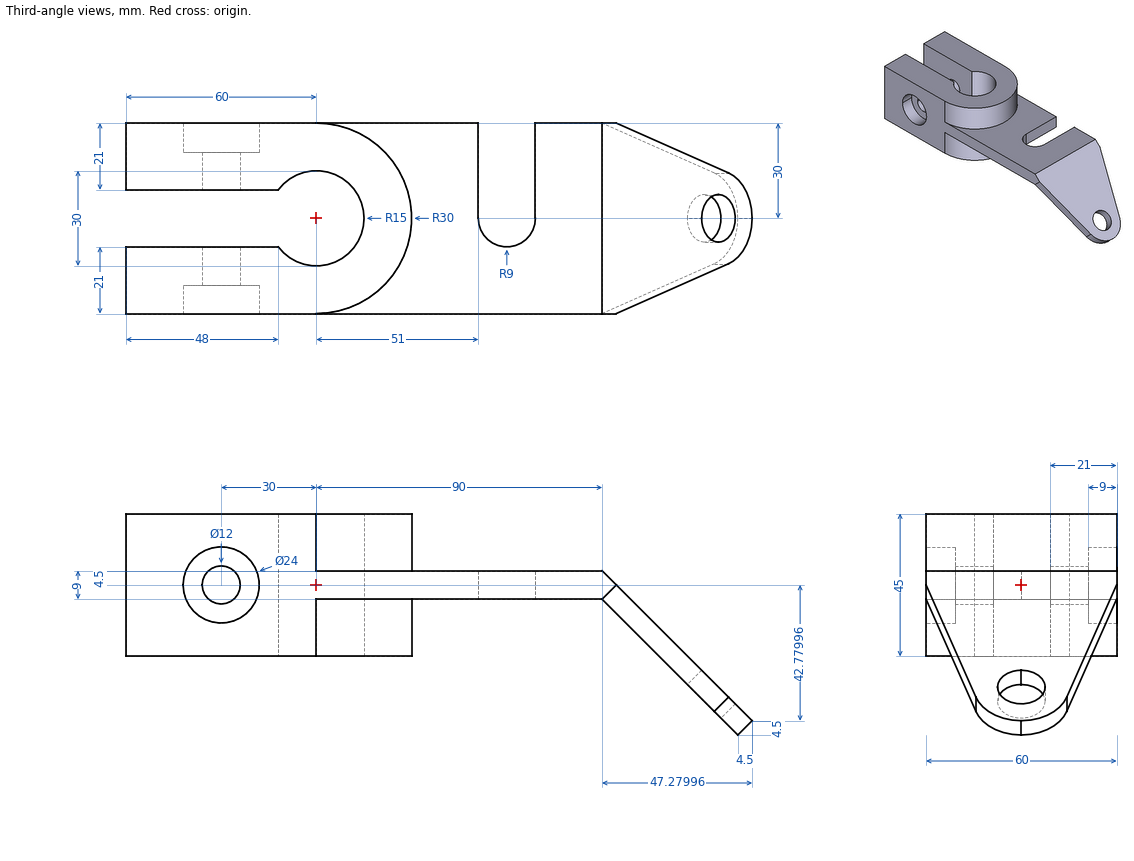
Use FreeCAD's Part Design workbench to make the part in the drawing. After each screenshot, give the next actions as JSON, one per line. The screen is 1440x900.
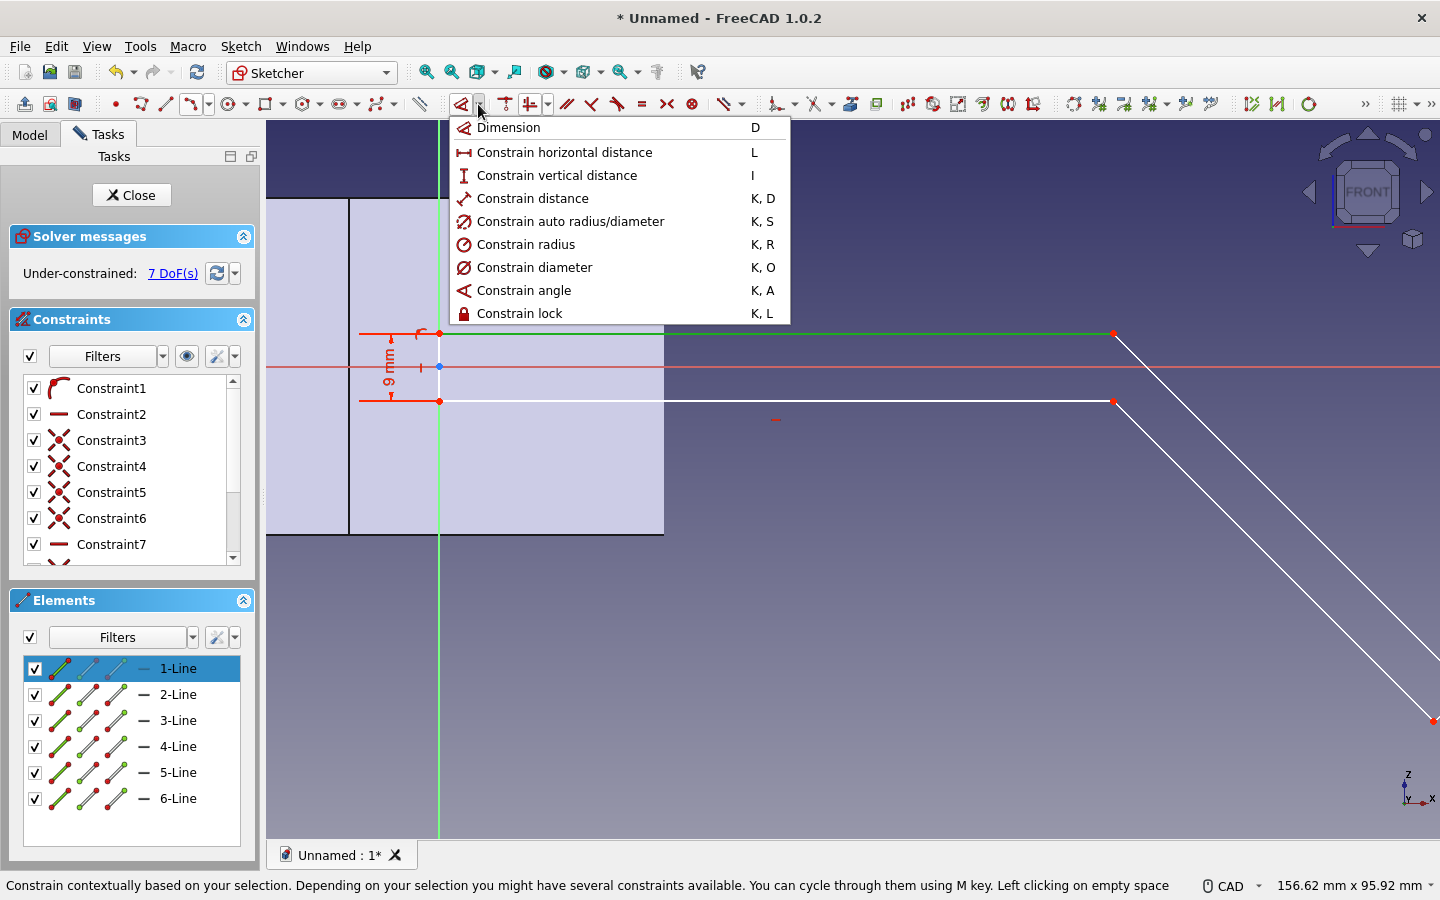
{"action": "left_click", "coordinate": [620, 152]}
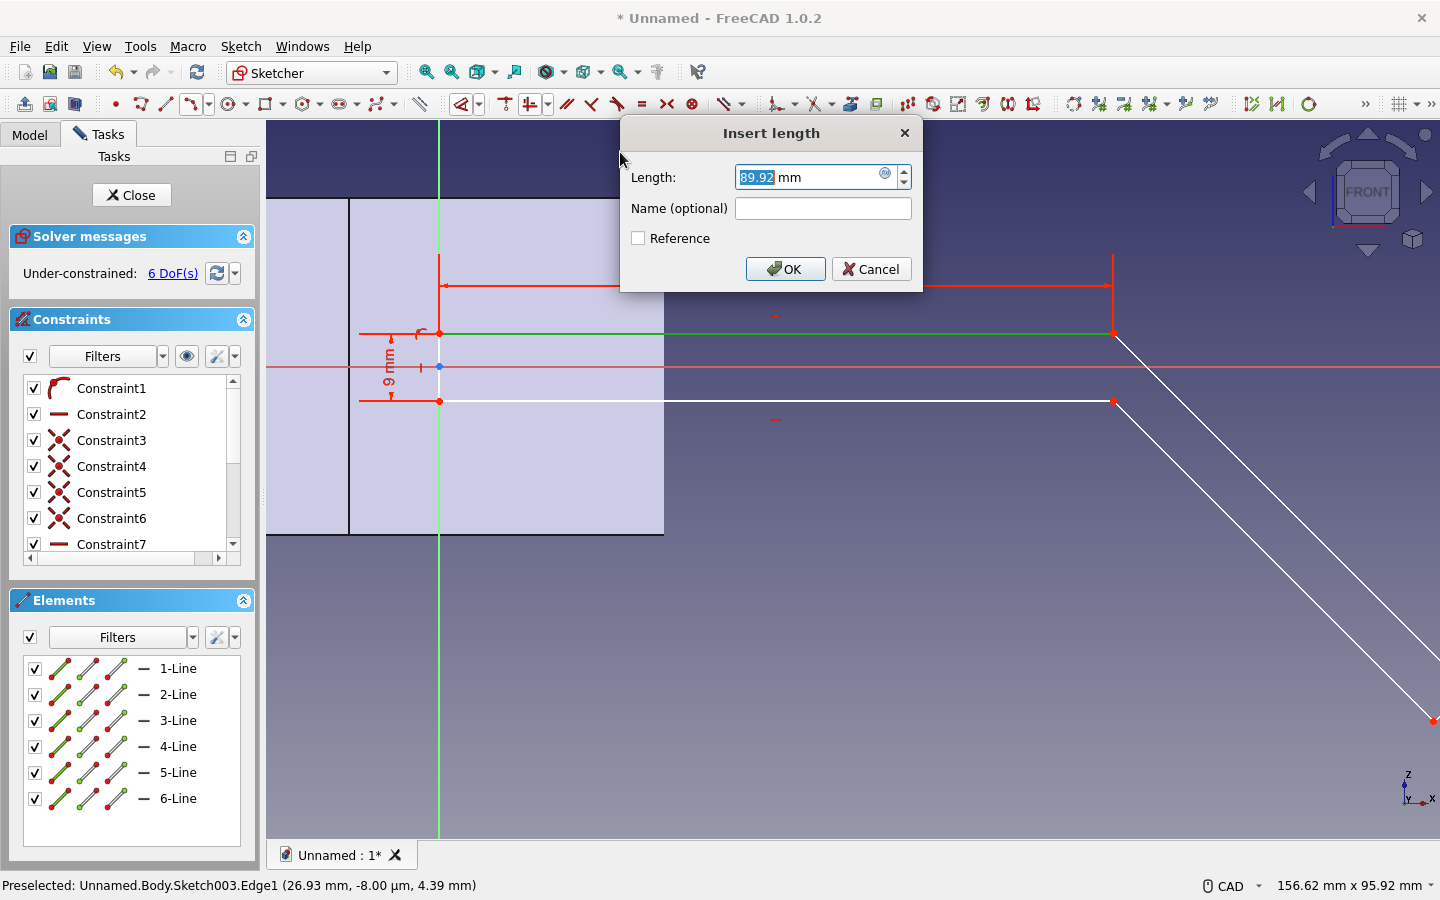
{"action": "type", "text": "90"}
{"action": "key", "text": "Return"}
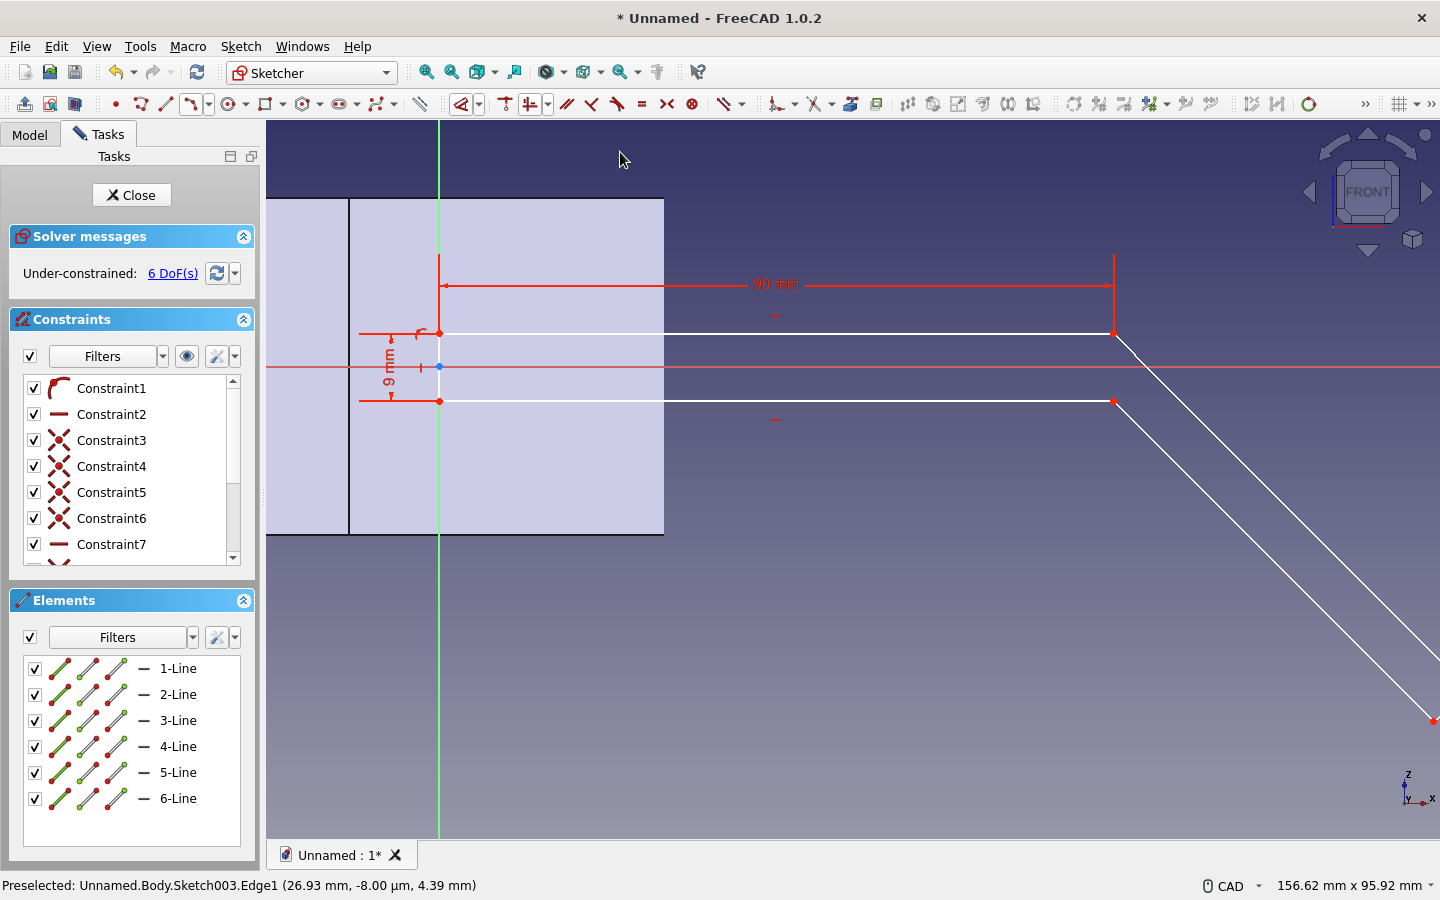
{"action": "left_click", "coordinate": [911, 401]}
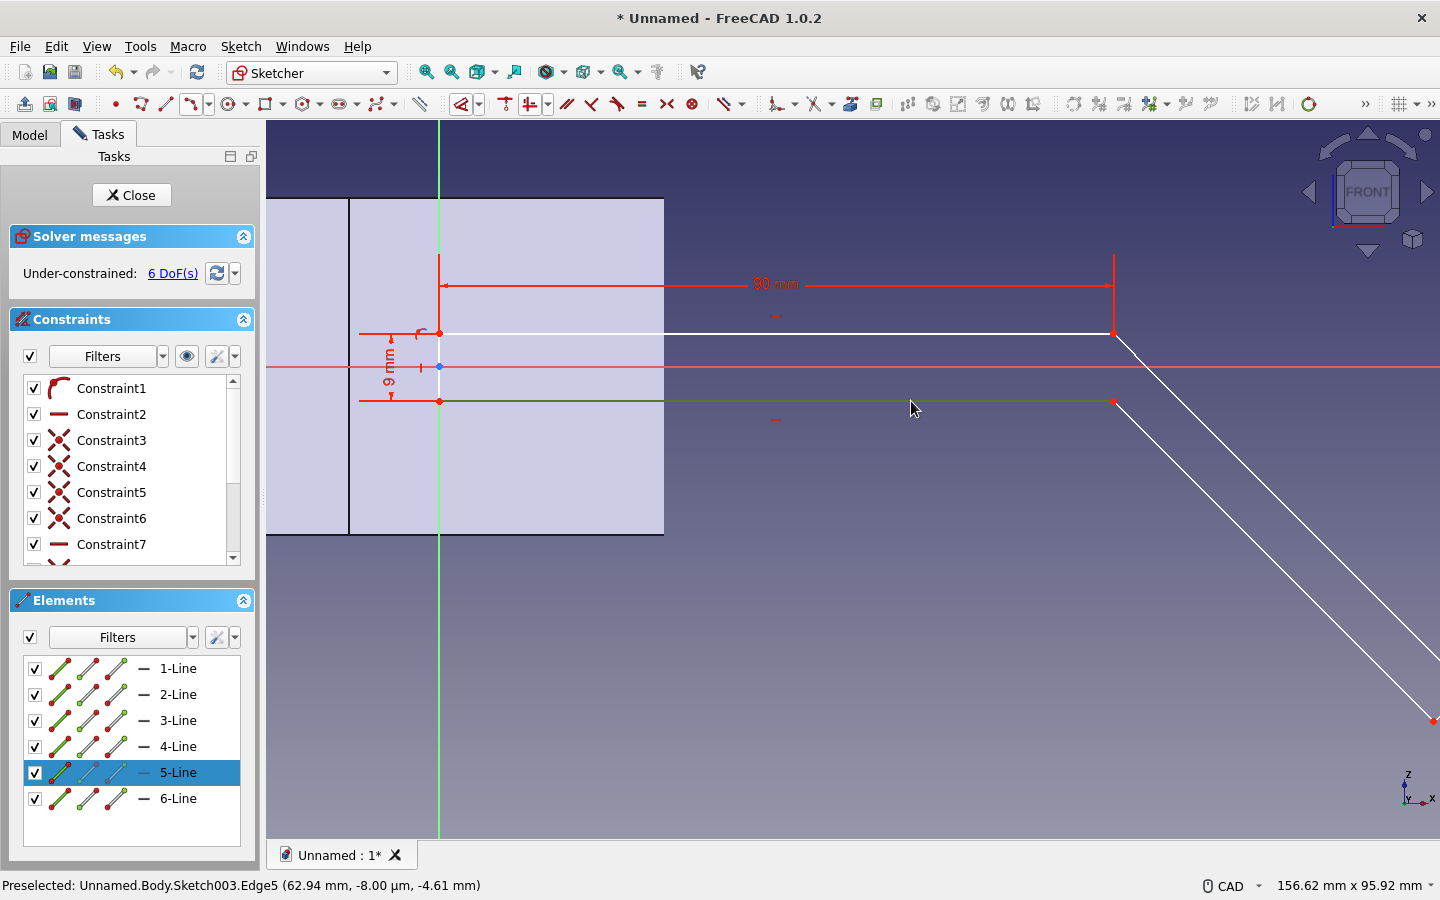
{"action": "left_click", "coordinate": [478, 104]}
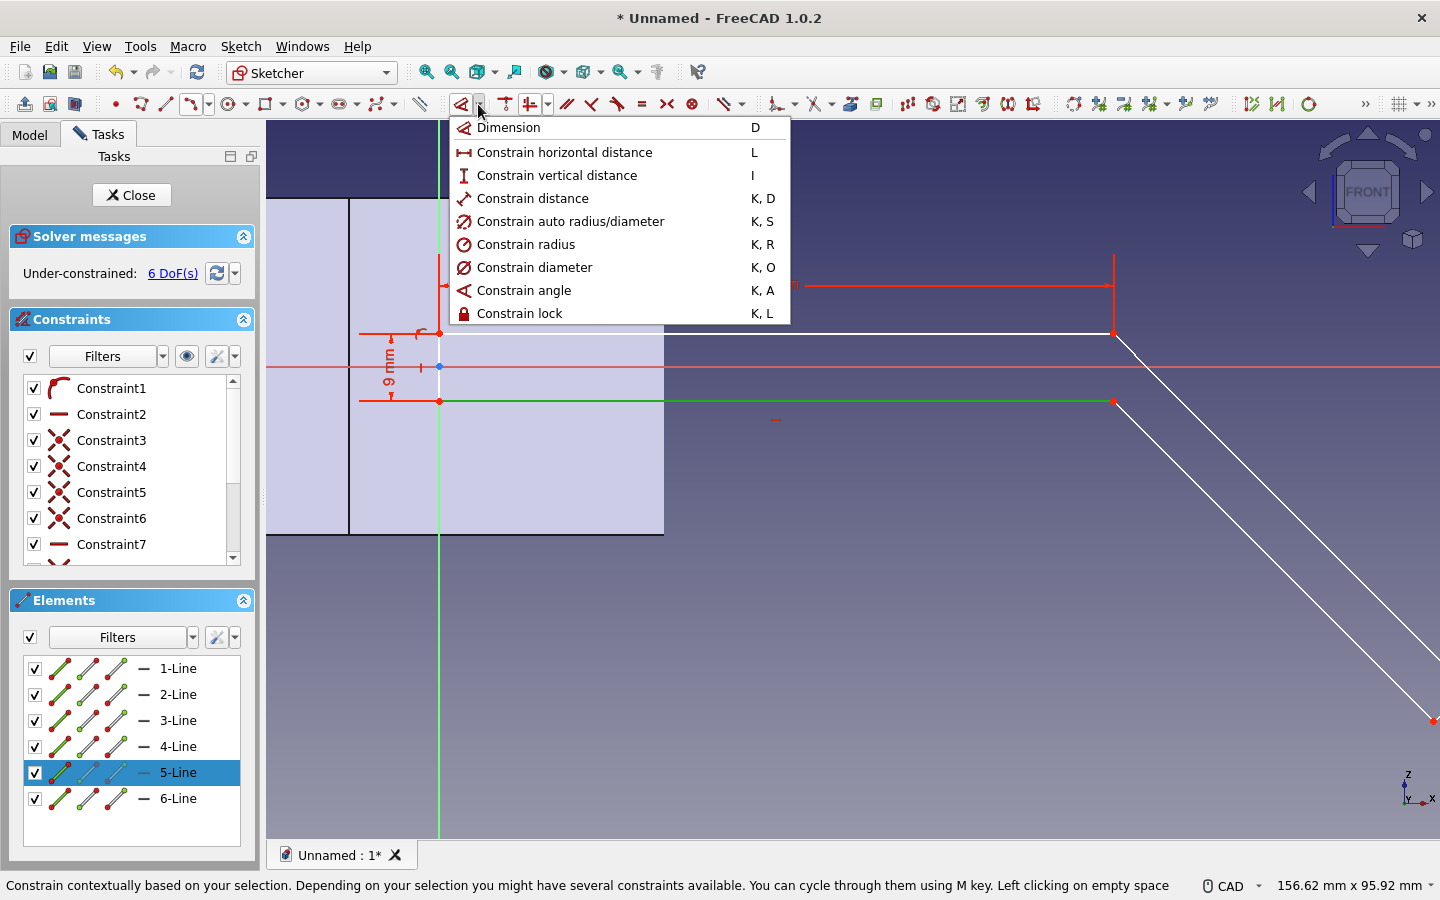
{"action": "left_click", "coordinate": [620, 152]}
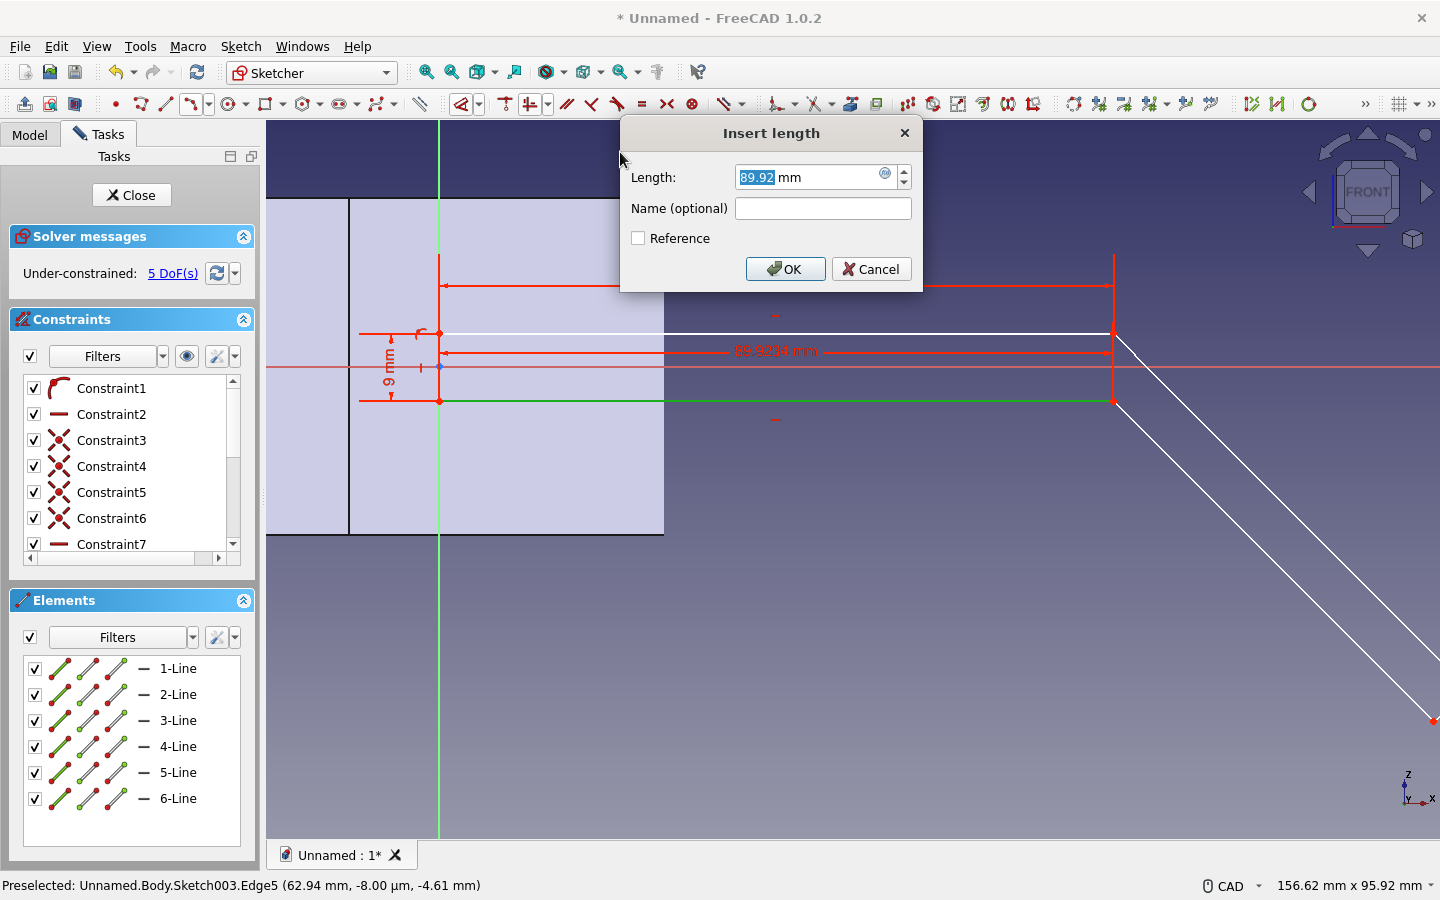
{"action": "type", "text": "90"}
{"action": "key", "text": "Return"}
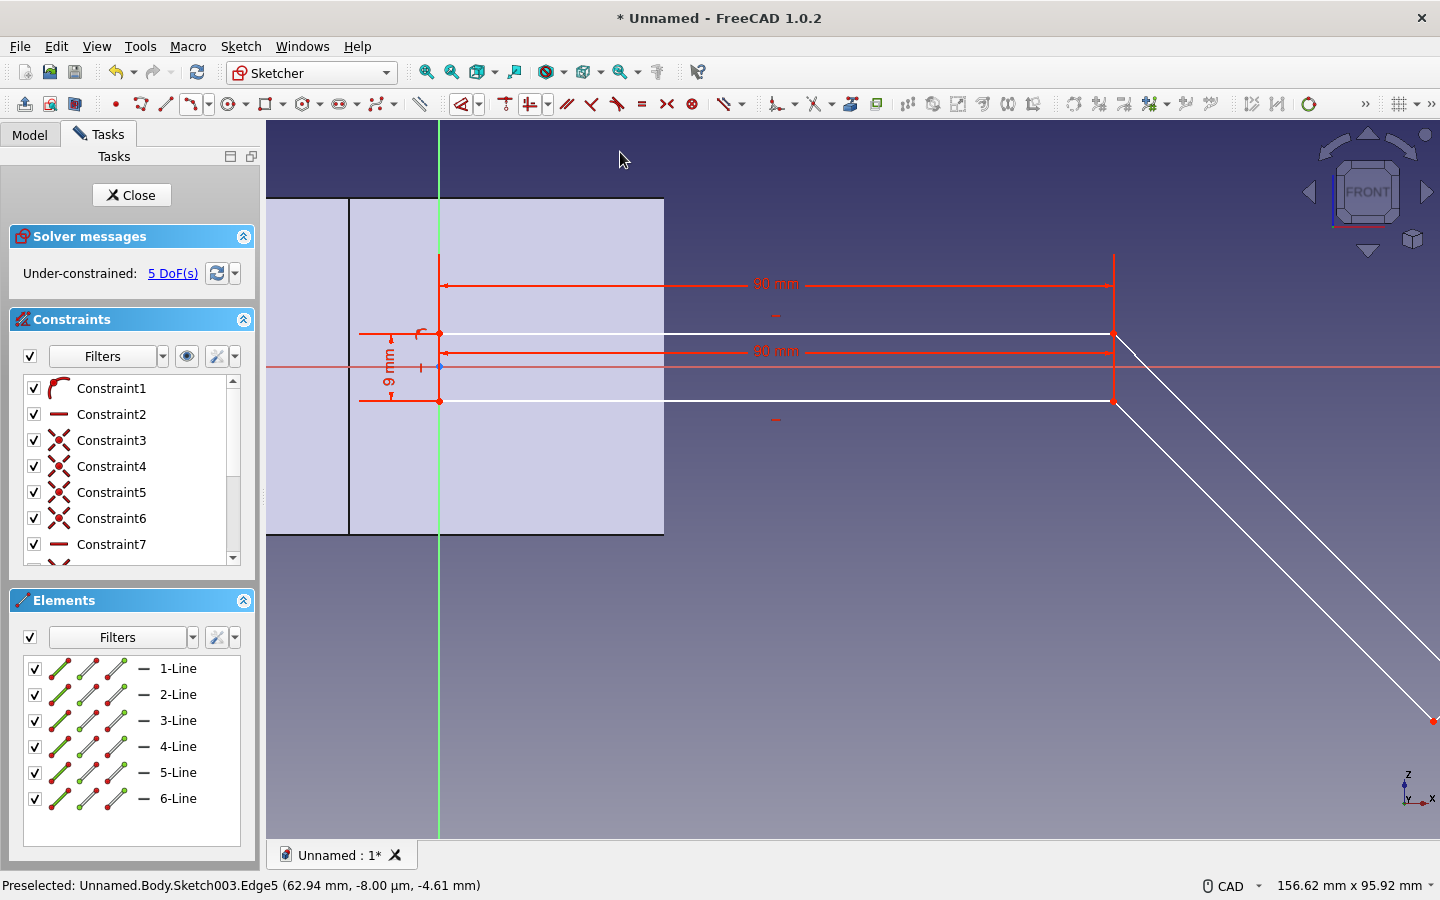
{"action": "left_click", "coordinate": [439, 334]}